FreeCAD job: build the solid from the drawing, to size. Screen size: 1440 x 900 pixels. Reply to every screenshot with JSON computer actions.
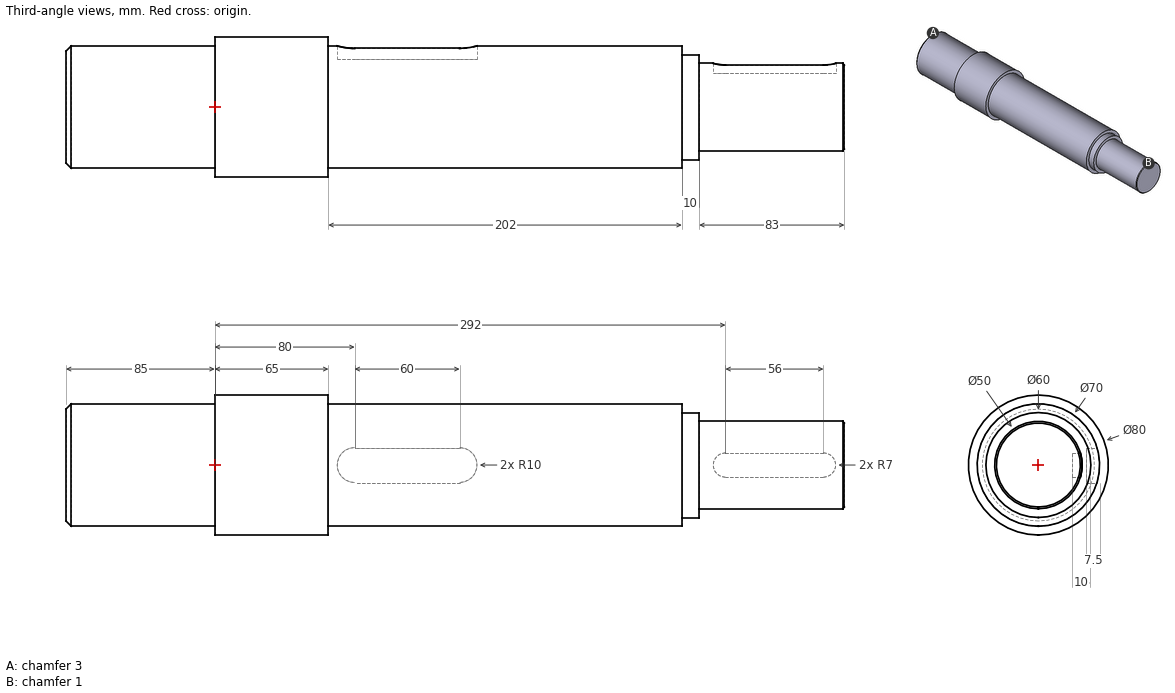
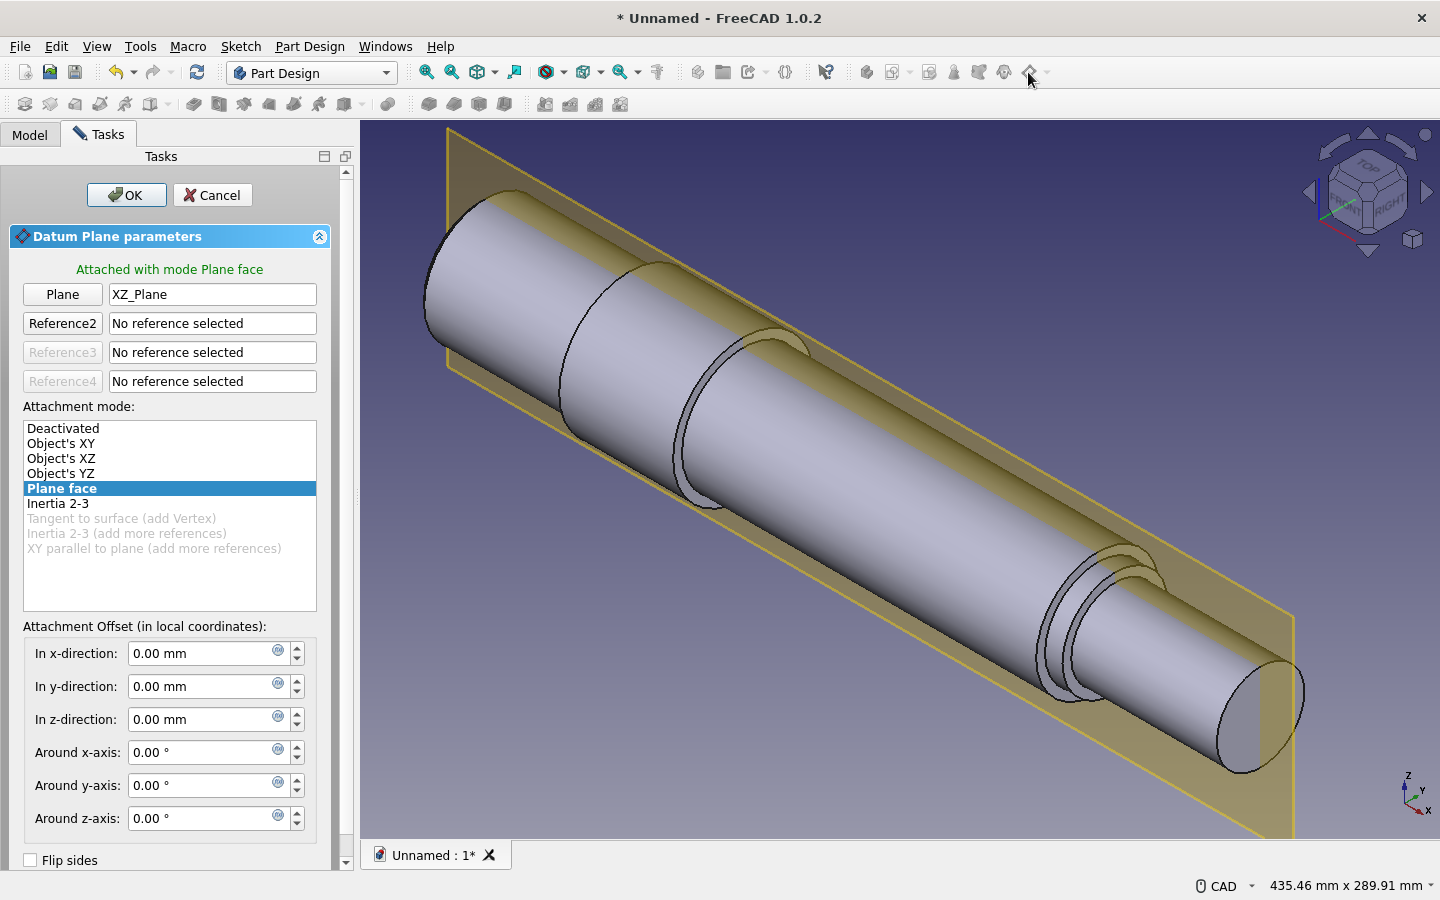
{"action": "triple_click", "coordinate": [210, 720]}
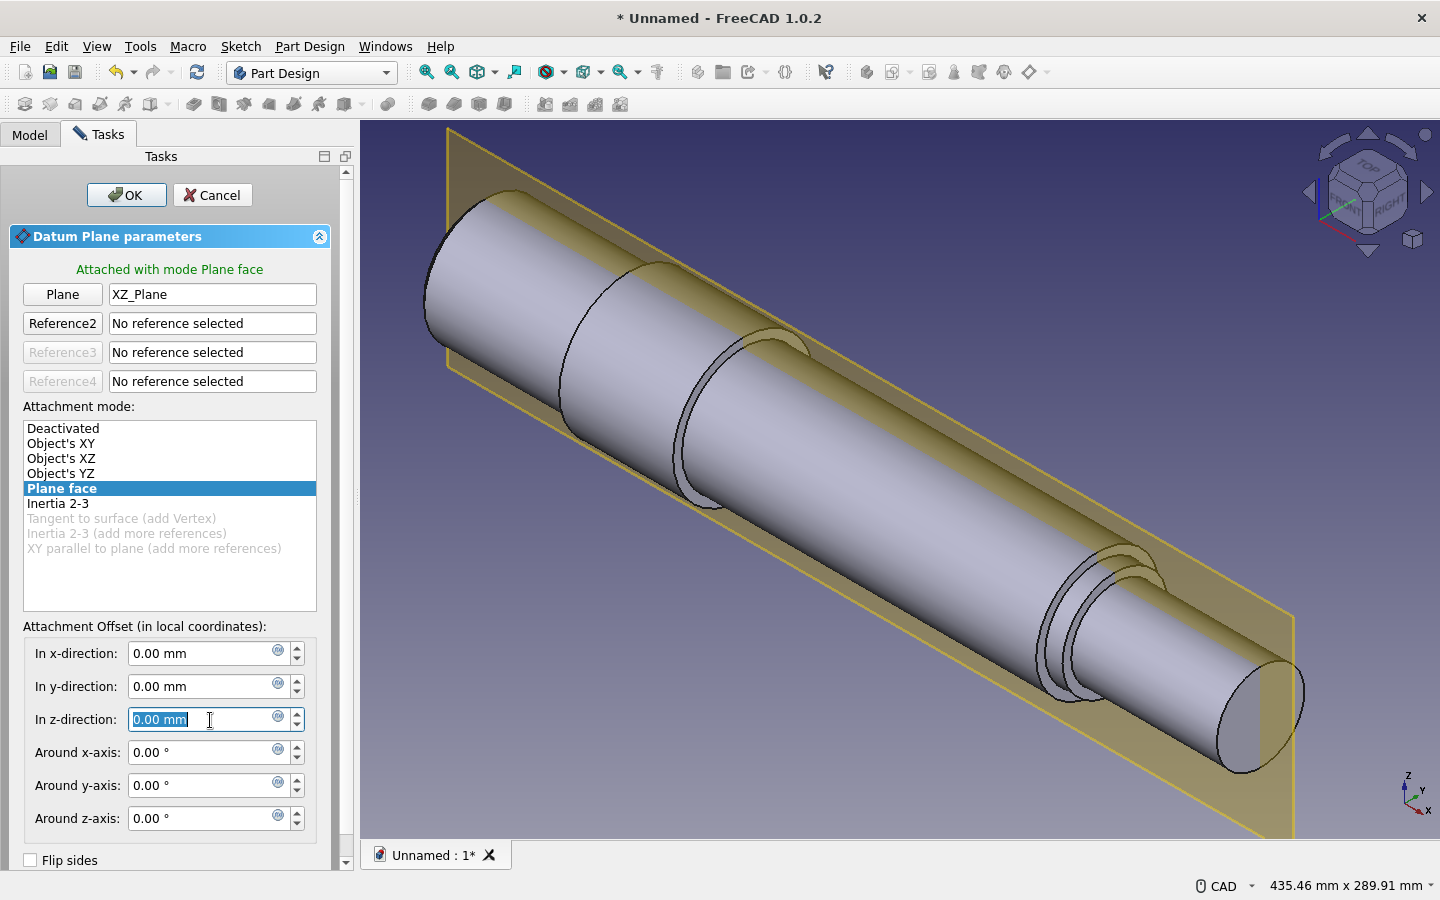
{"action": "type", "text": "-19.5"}
{"action": "key", "text": "Tab"}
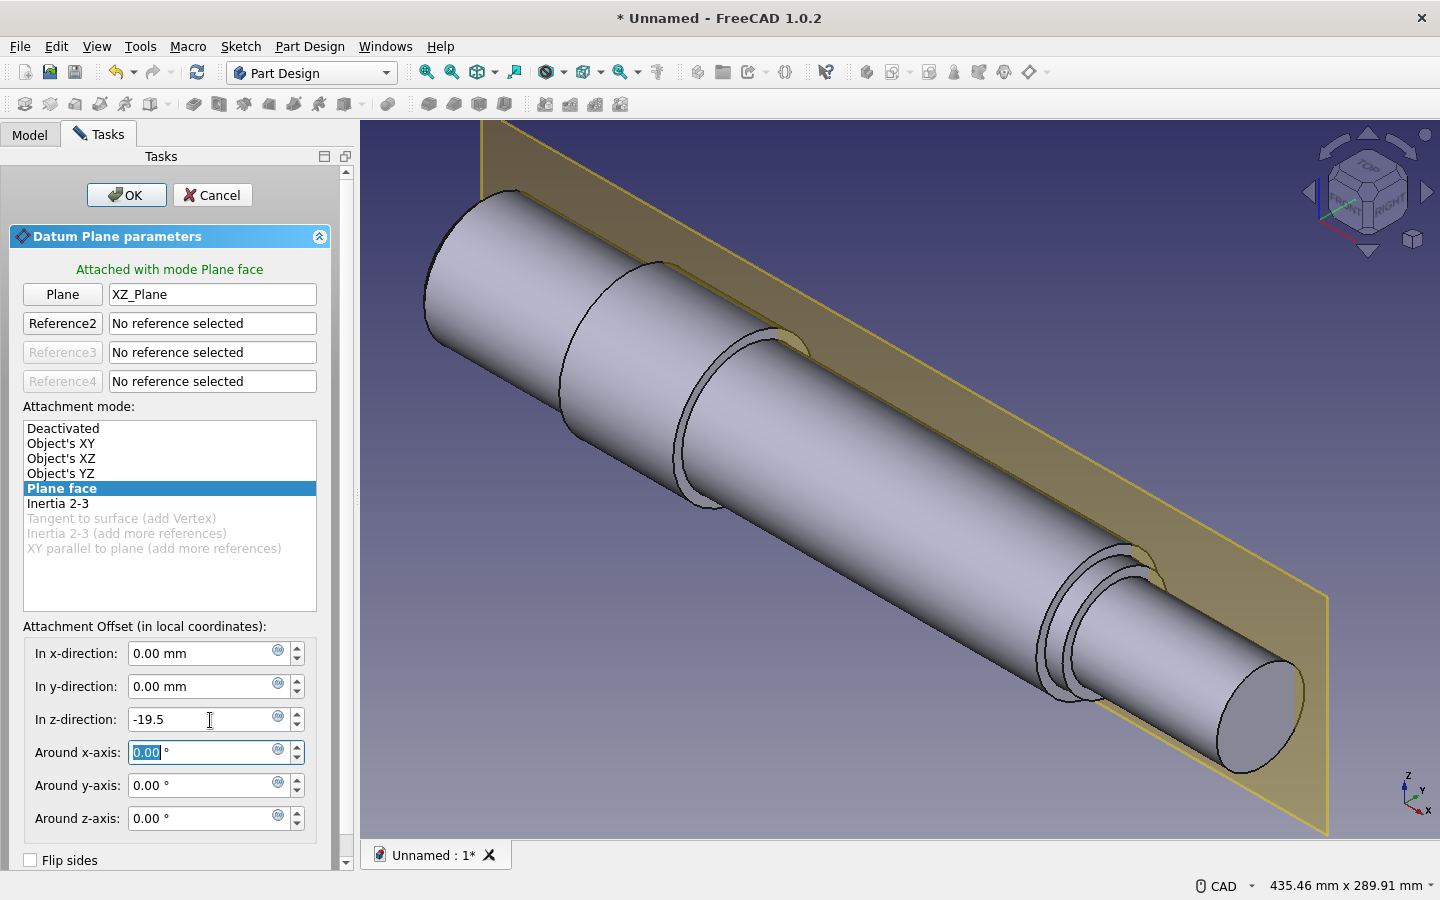
{"action": "left_click", "coordinate": [127, 195]}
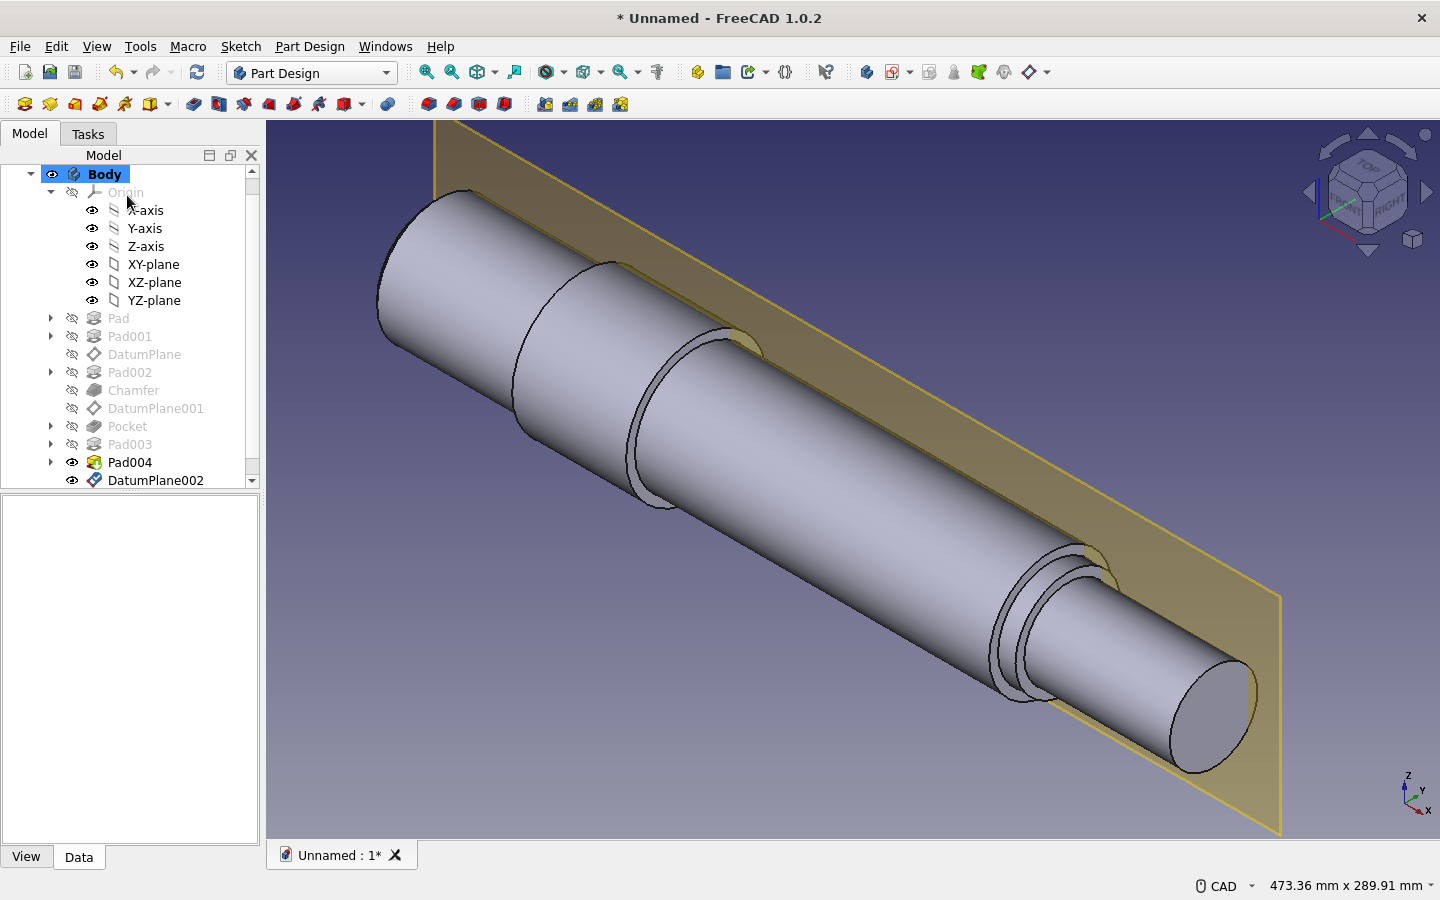
{"action": "left_click", "coordinate": [117, 480]}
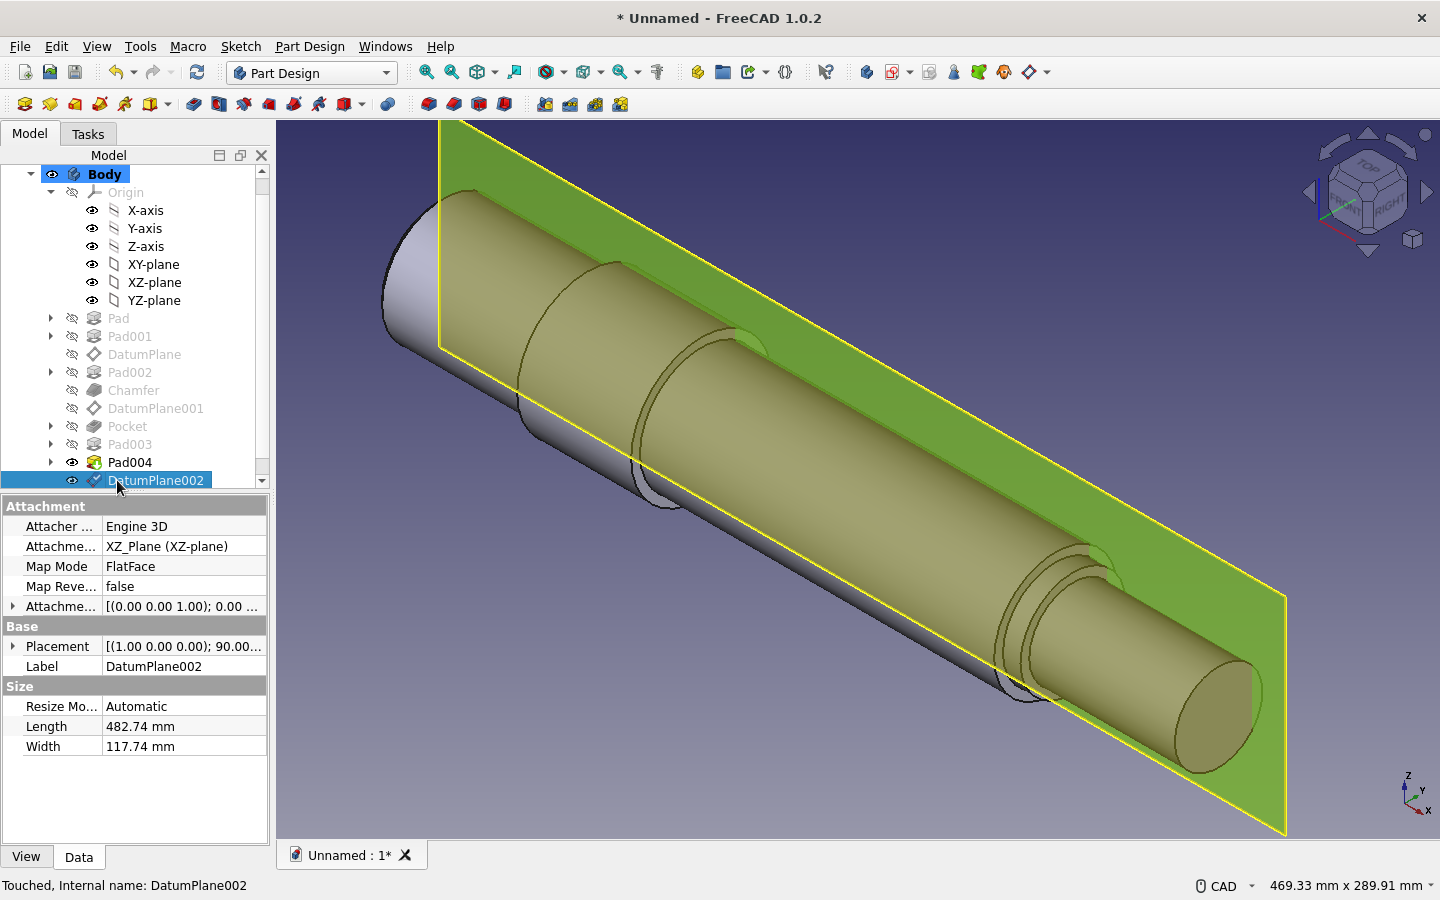
{"action": "left_click", "coordinate": [892, 72]}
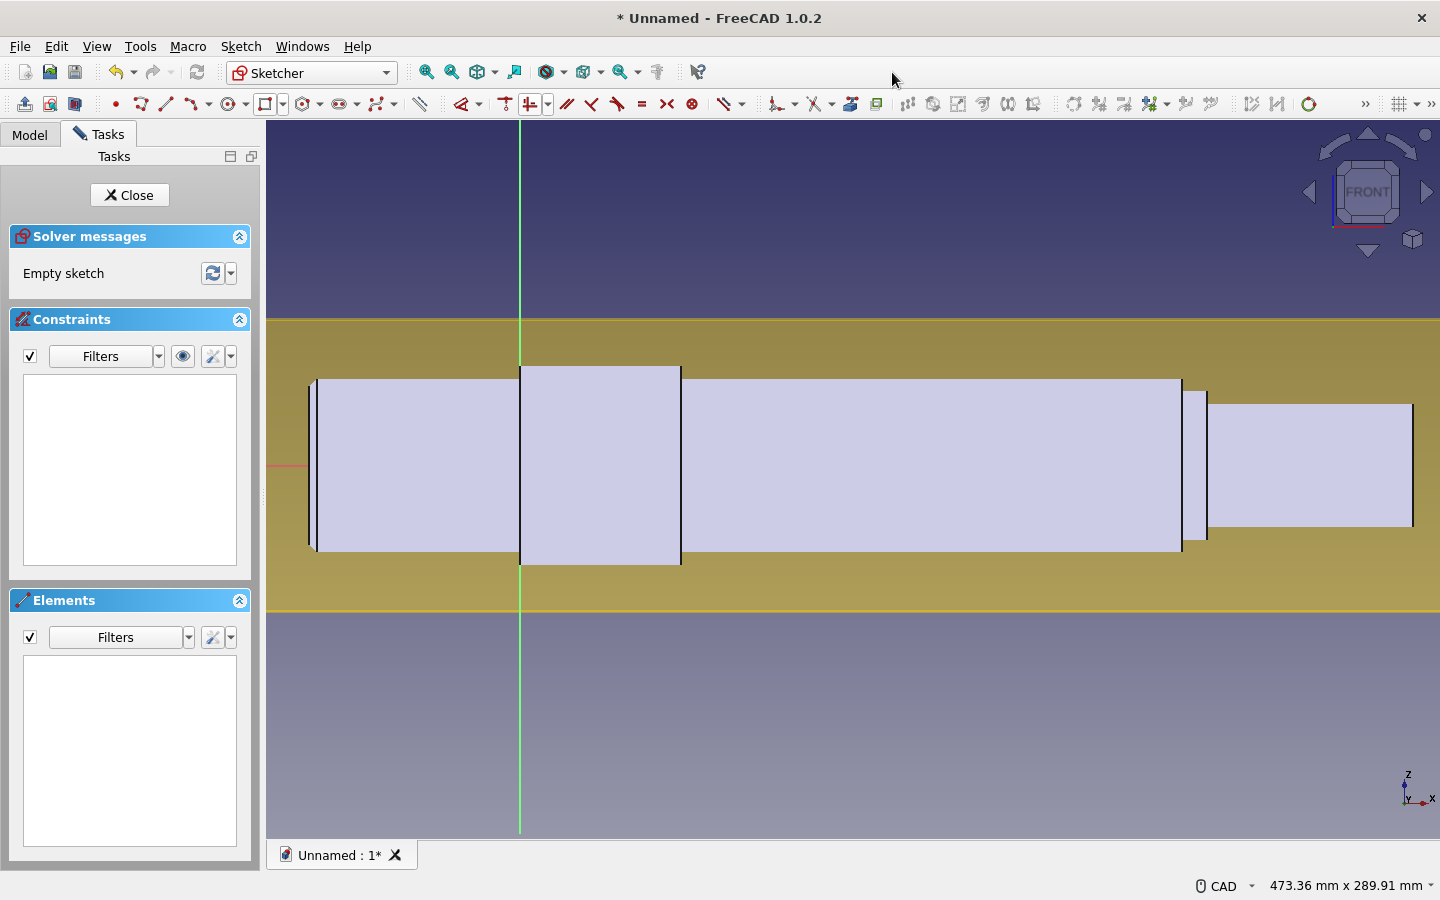
{"action": "key", "text": "q s"}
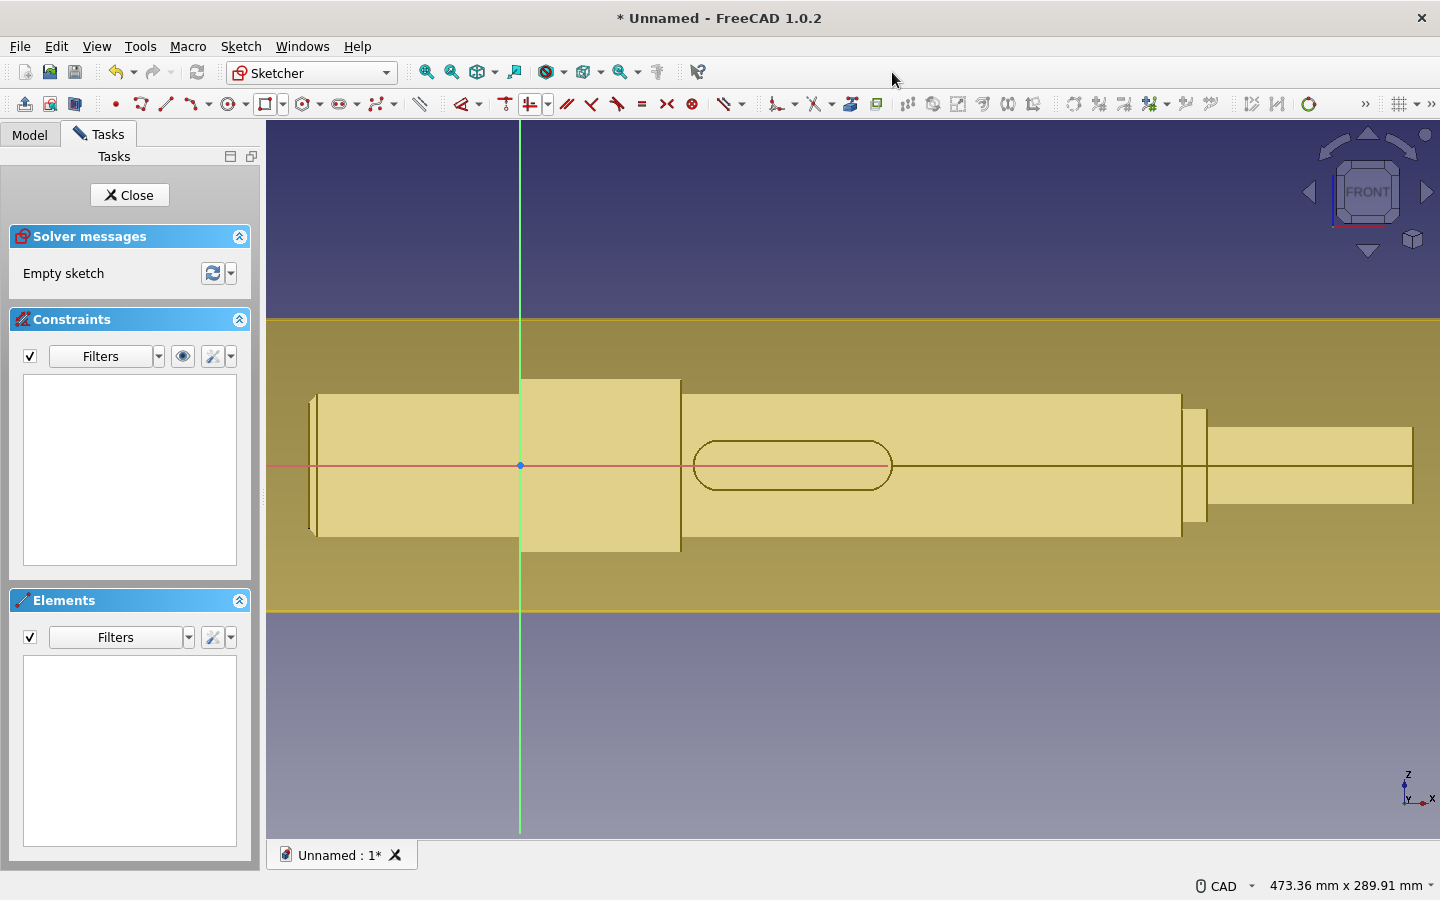
{"action": "scroll", "coordinate": [784, 480], "scroll_direction": "down", "scroll_amount": 5}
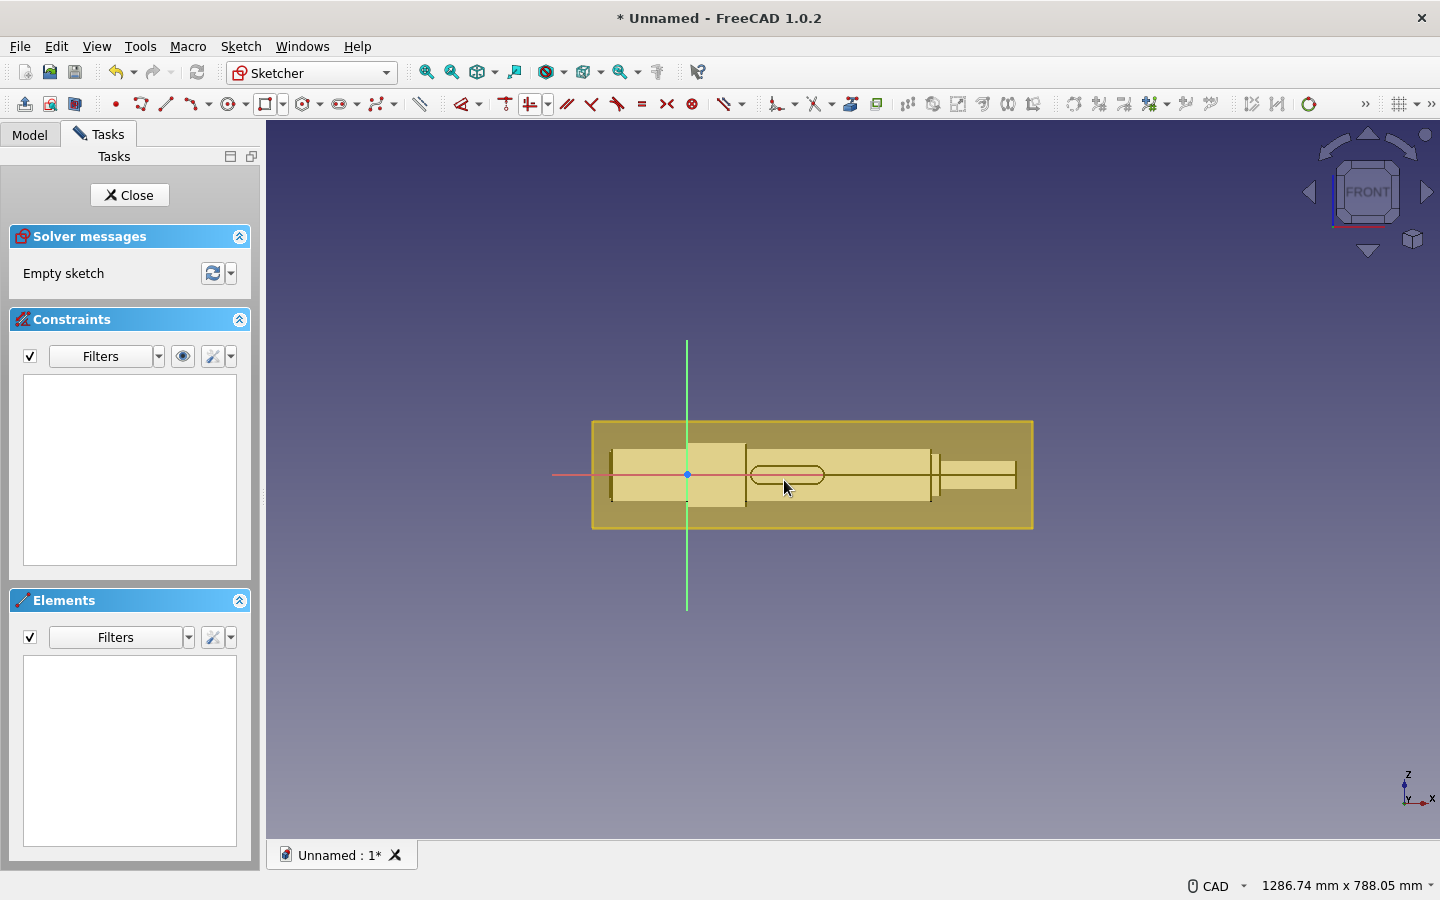
{"action": "scroll", "coordinate": [999, 475], "scroll_direction": "up", "scroll_amount": 12}